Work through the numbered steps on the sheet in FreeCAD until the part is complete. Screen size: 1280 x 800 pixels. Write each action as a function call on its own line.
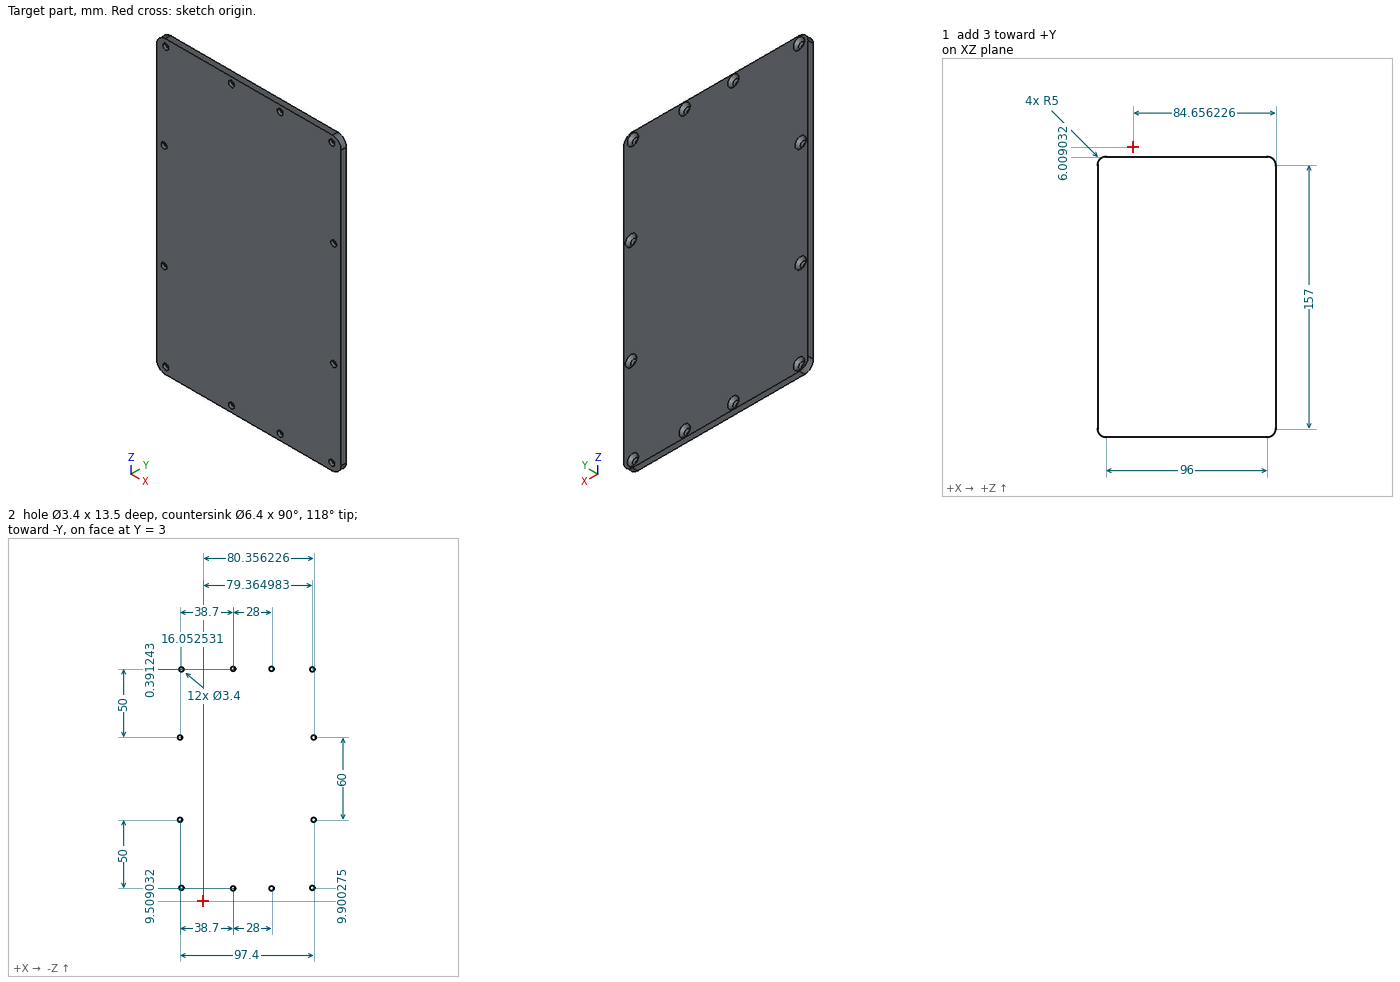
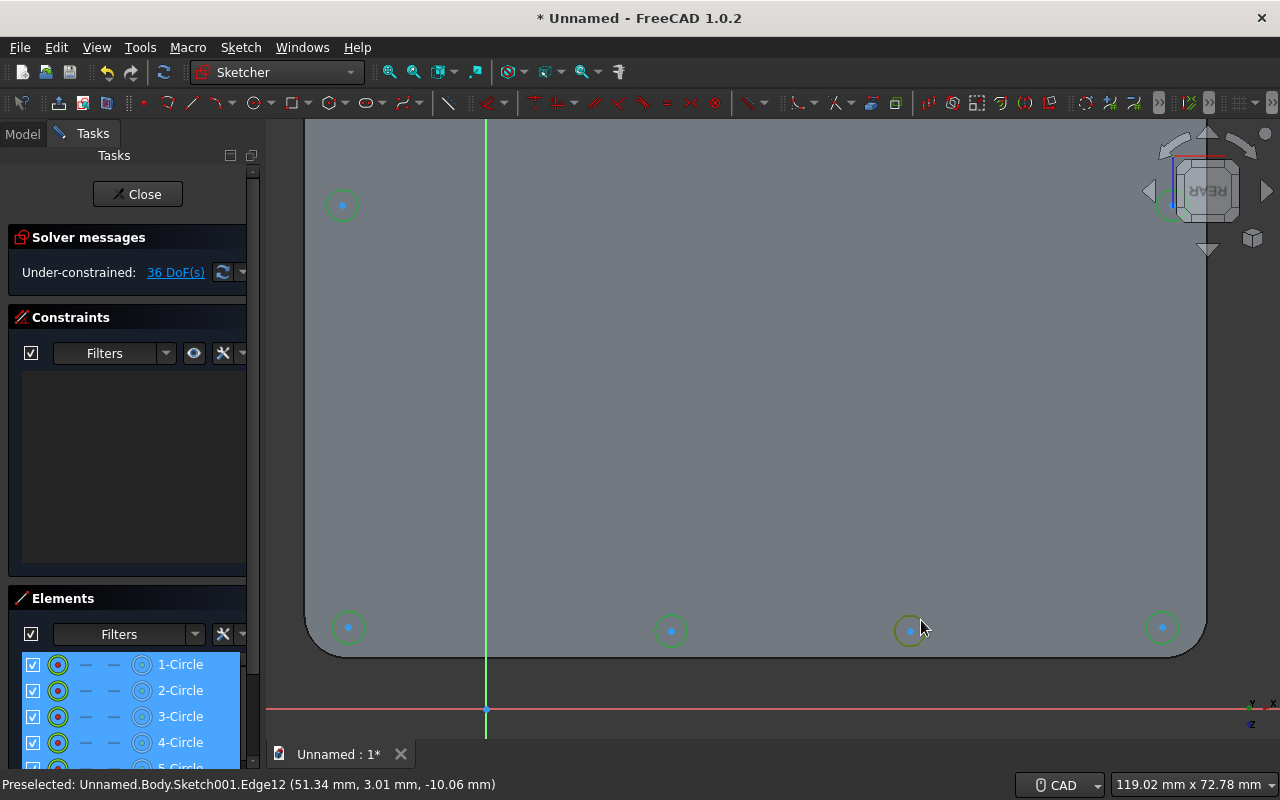
click(668, 104)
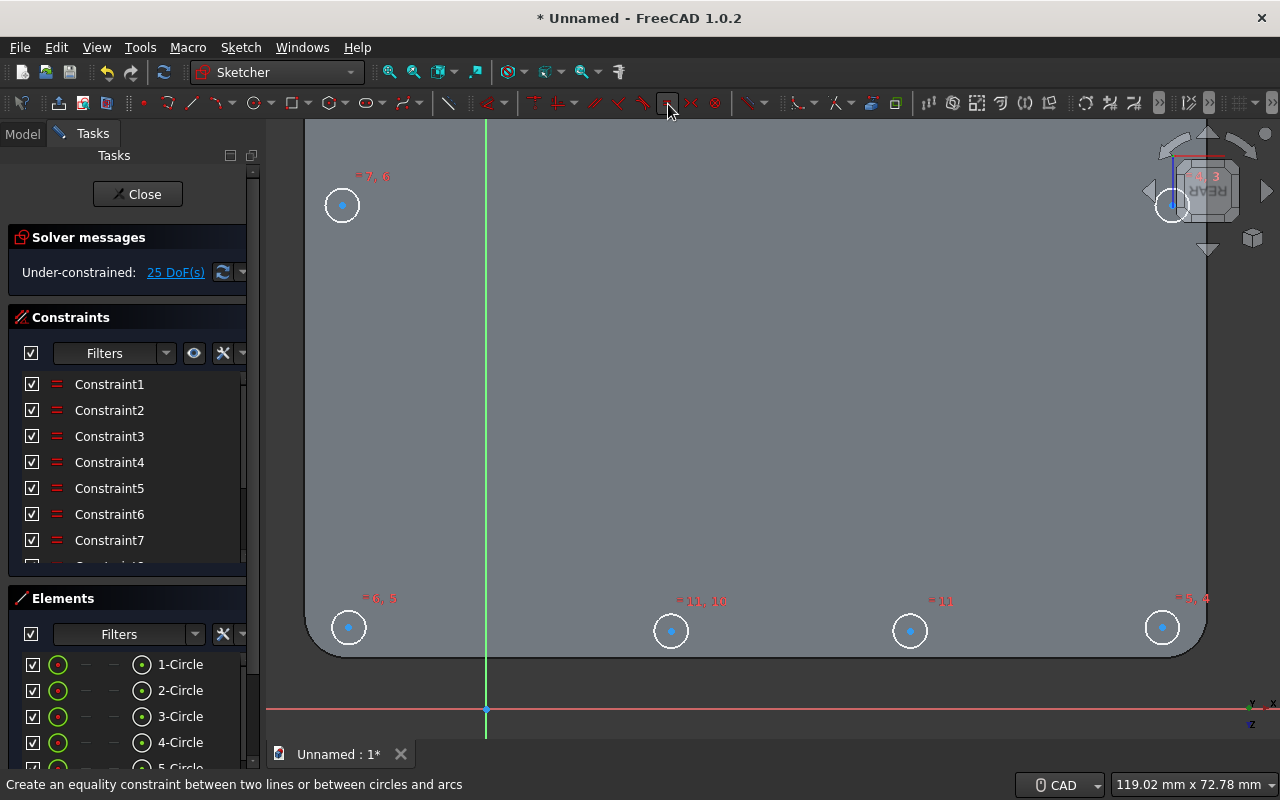
scroll(682, 622, down, 6)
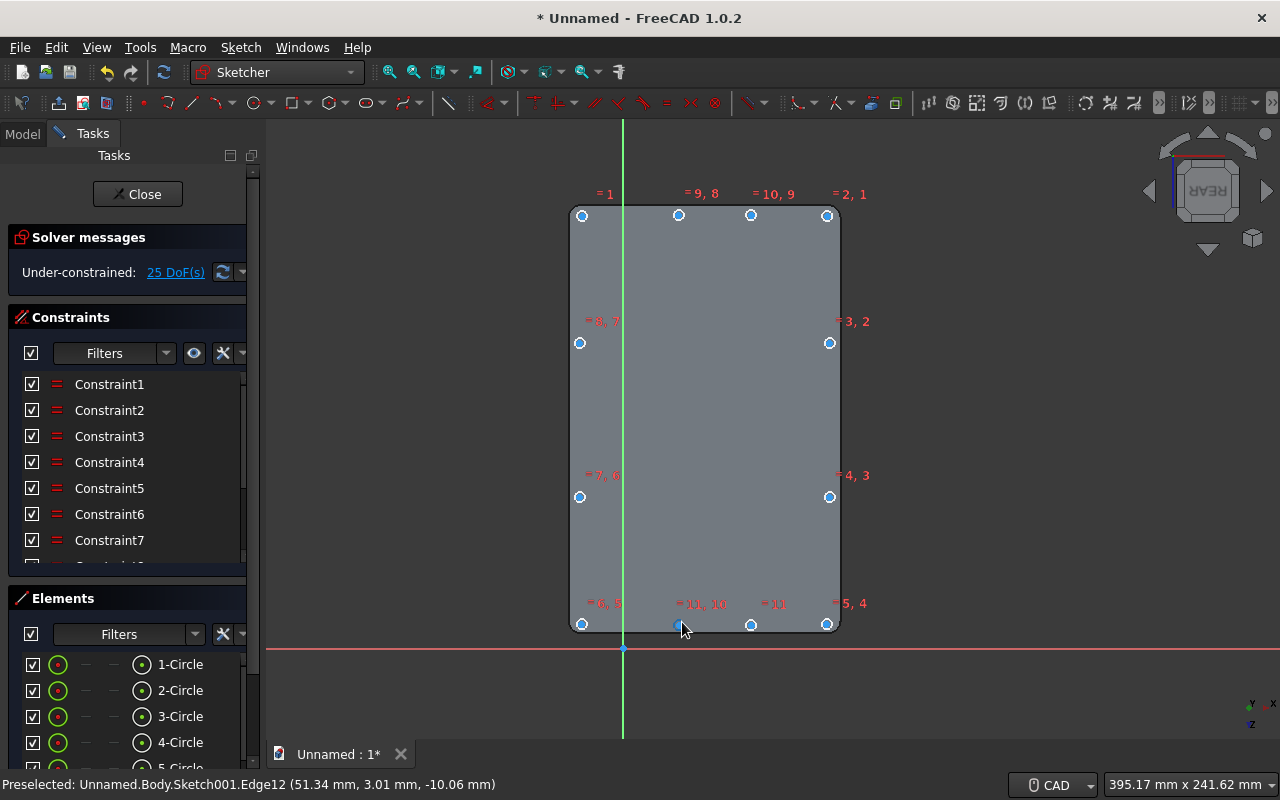
click(582, 216)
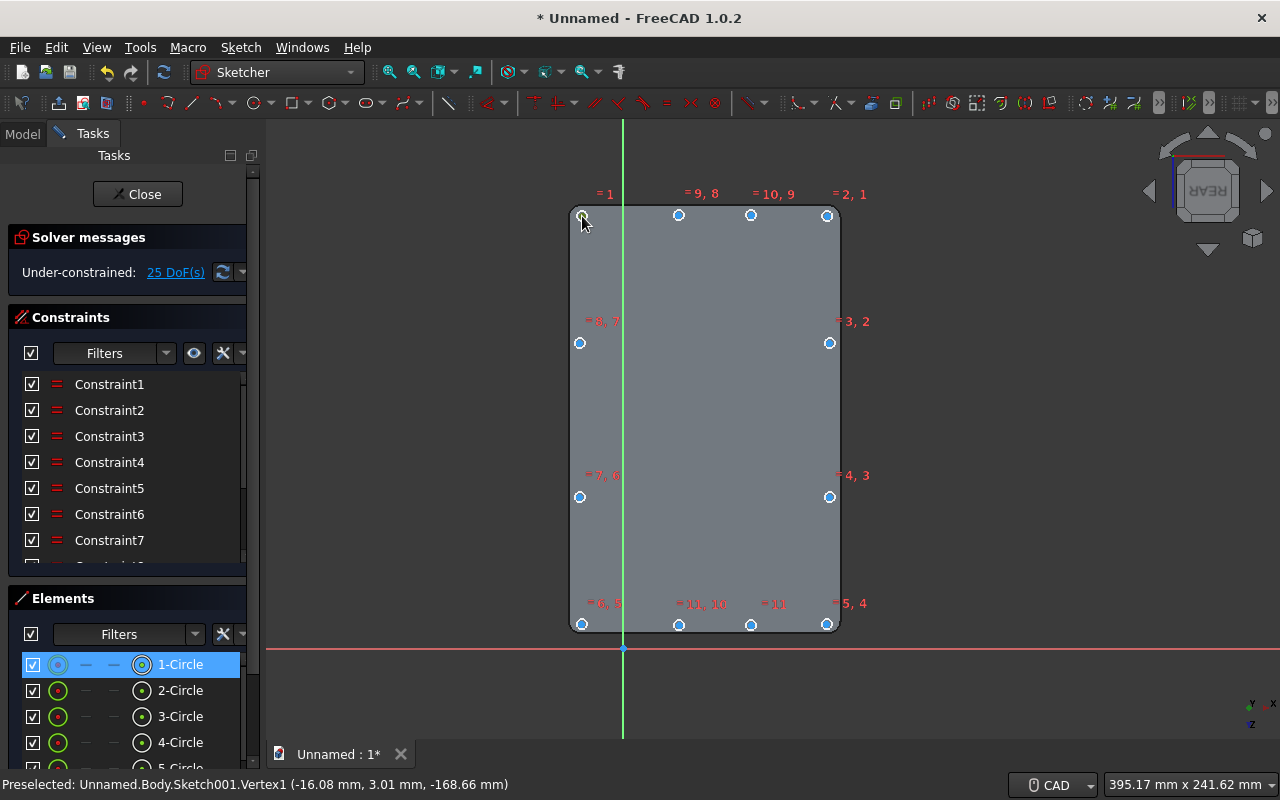
click(827, 216)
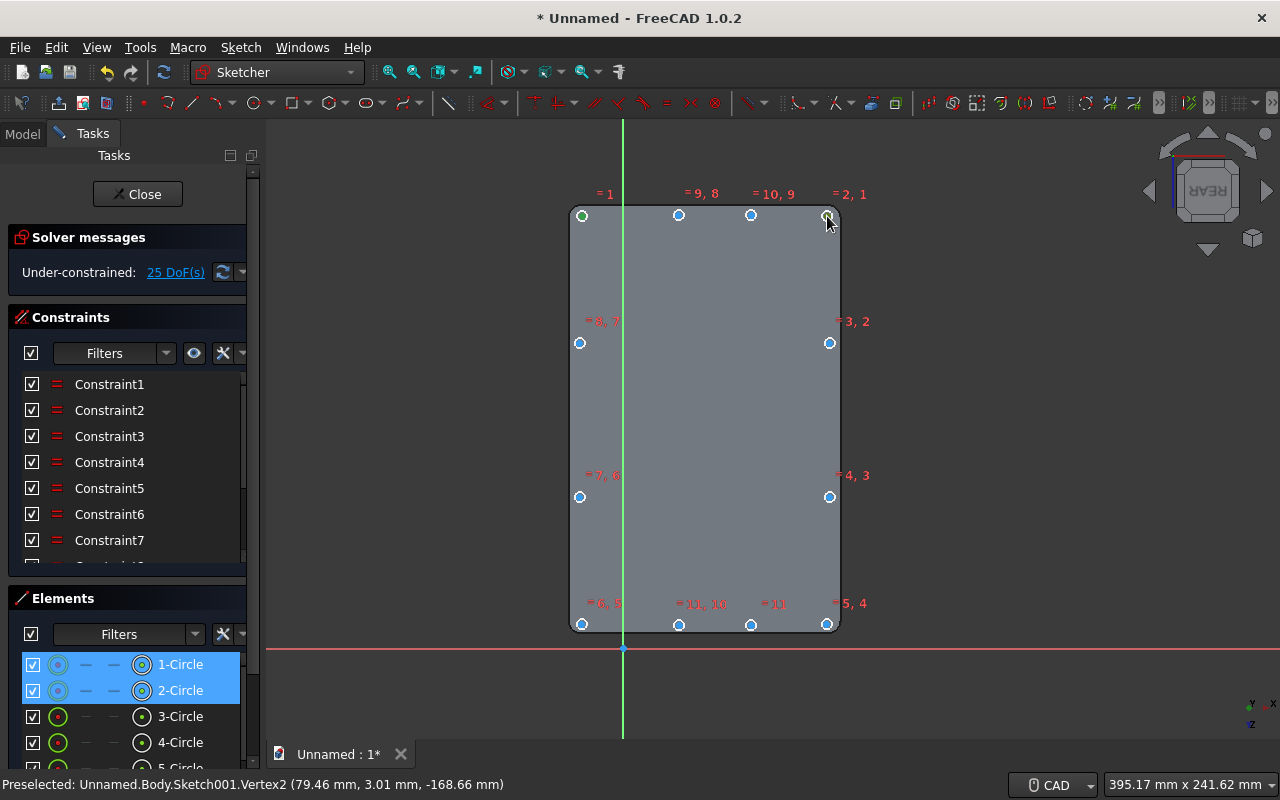
key(h)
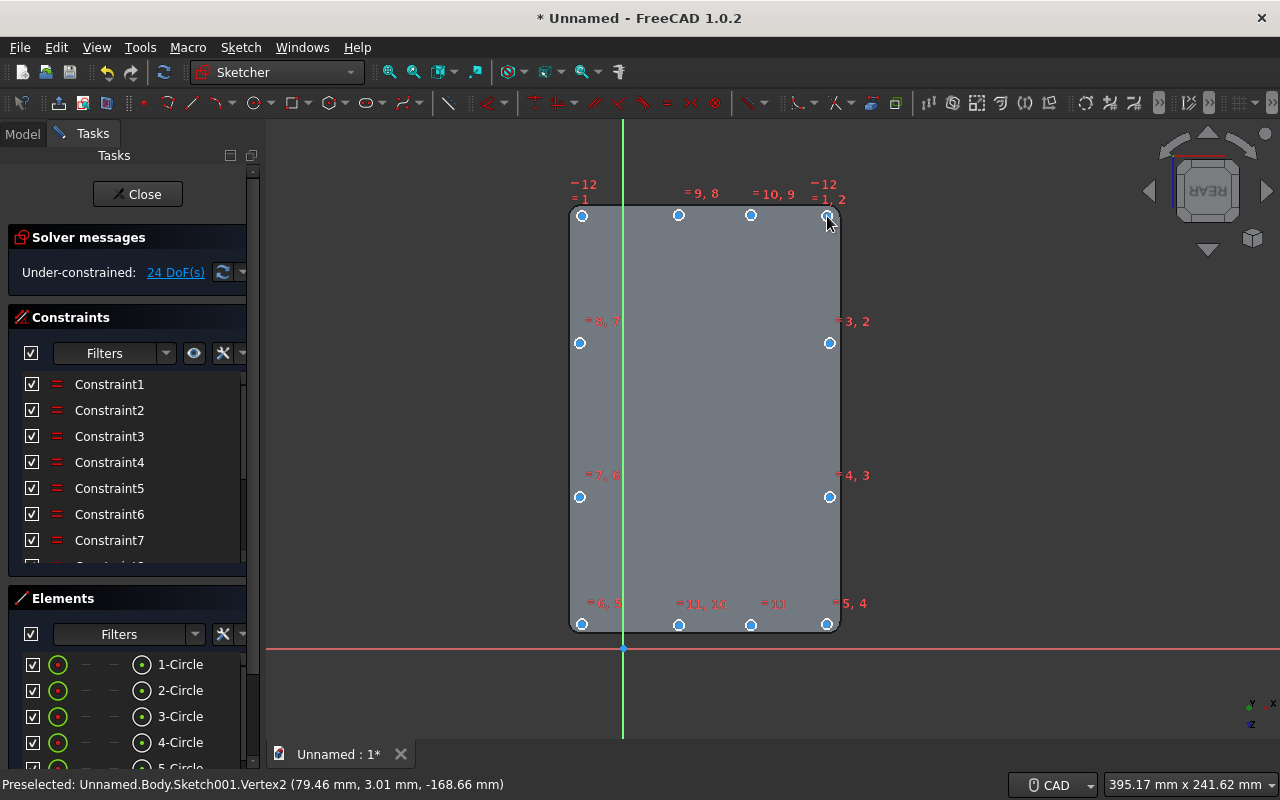
click(830, 343)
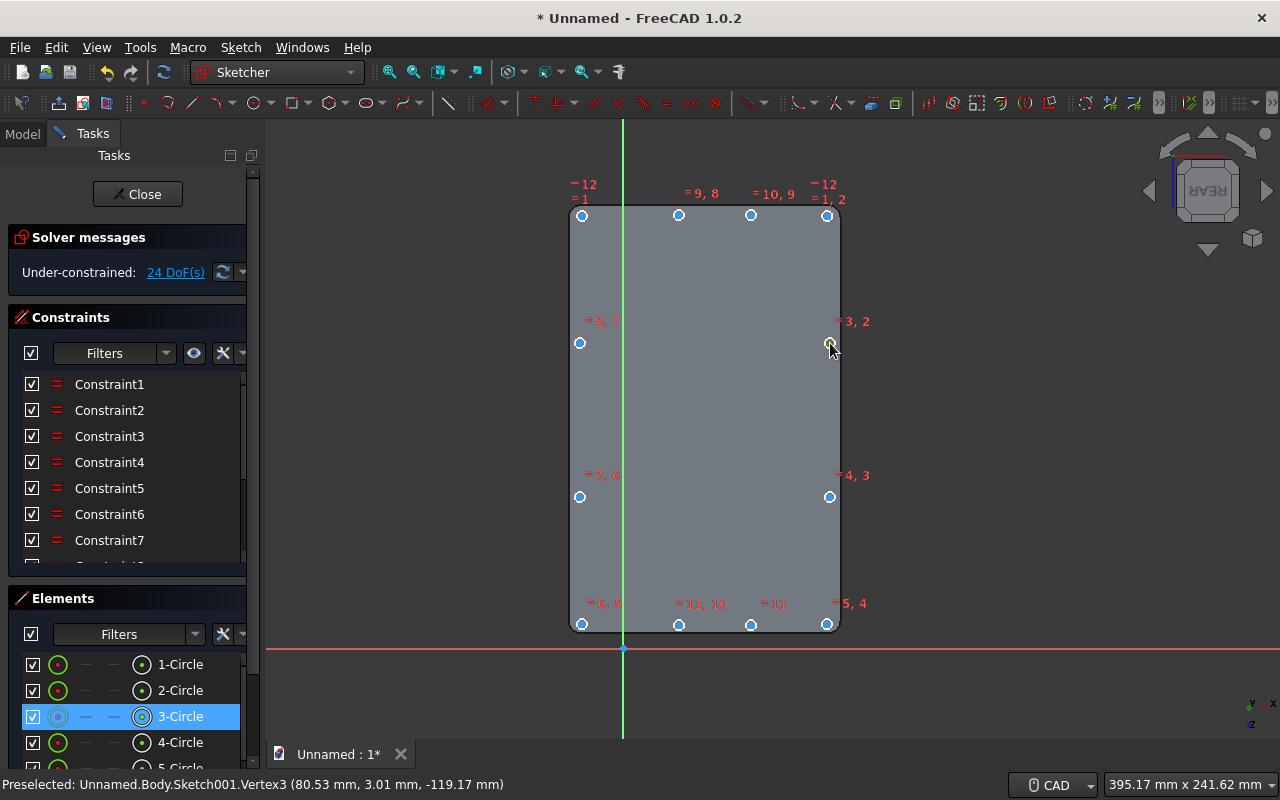
click(830, 497)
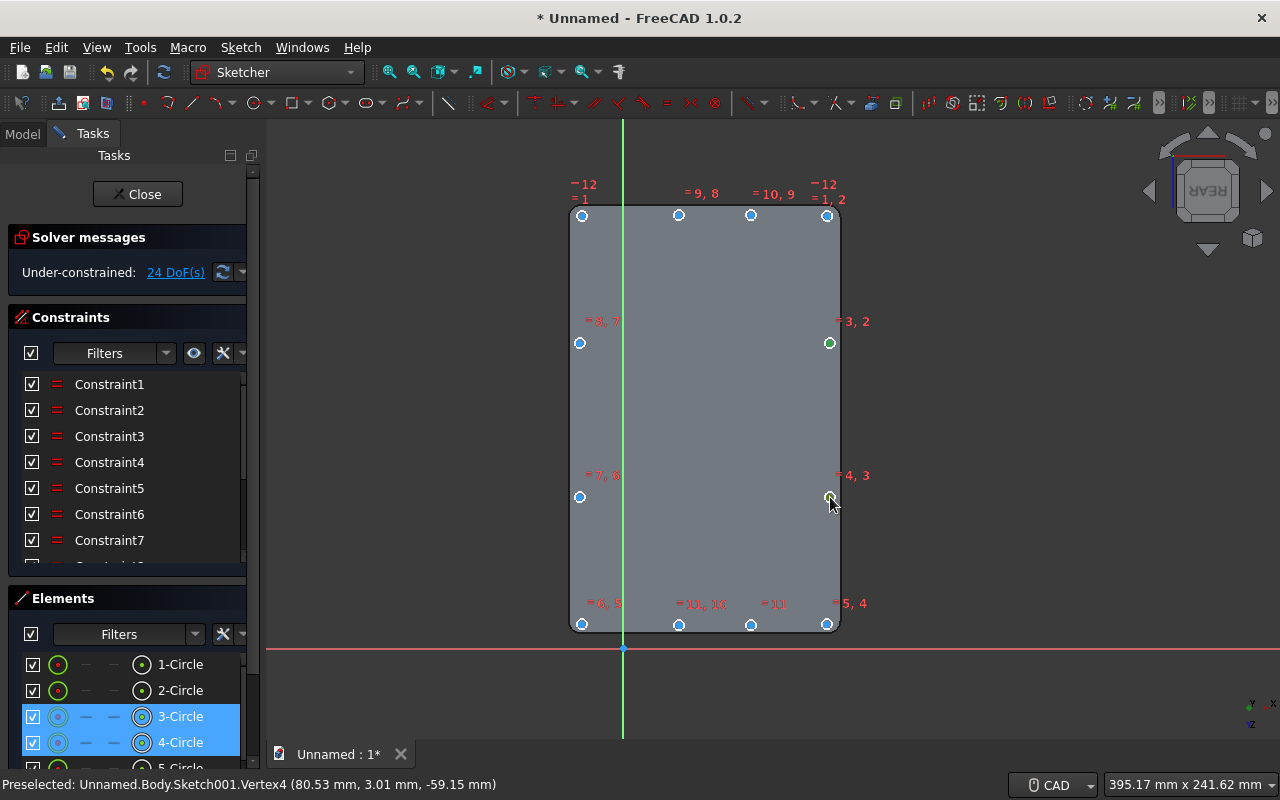
click(576, 104)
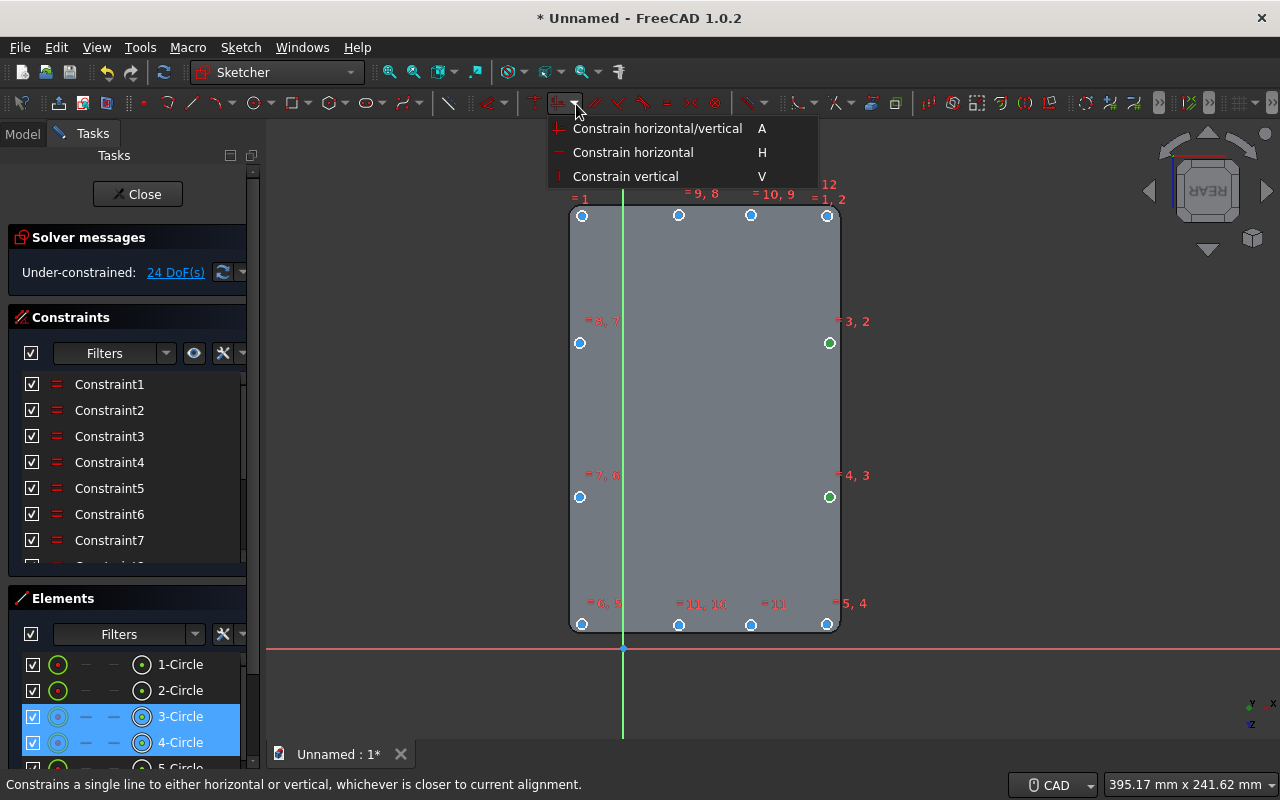
click(683, 176)